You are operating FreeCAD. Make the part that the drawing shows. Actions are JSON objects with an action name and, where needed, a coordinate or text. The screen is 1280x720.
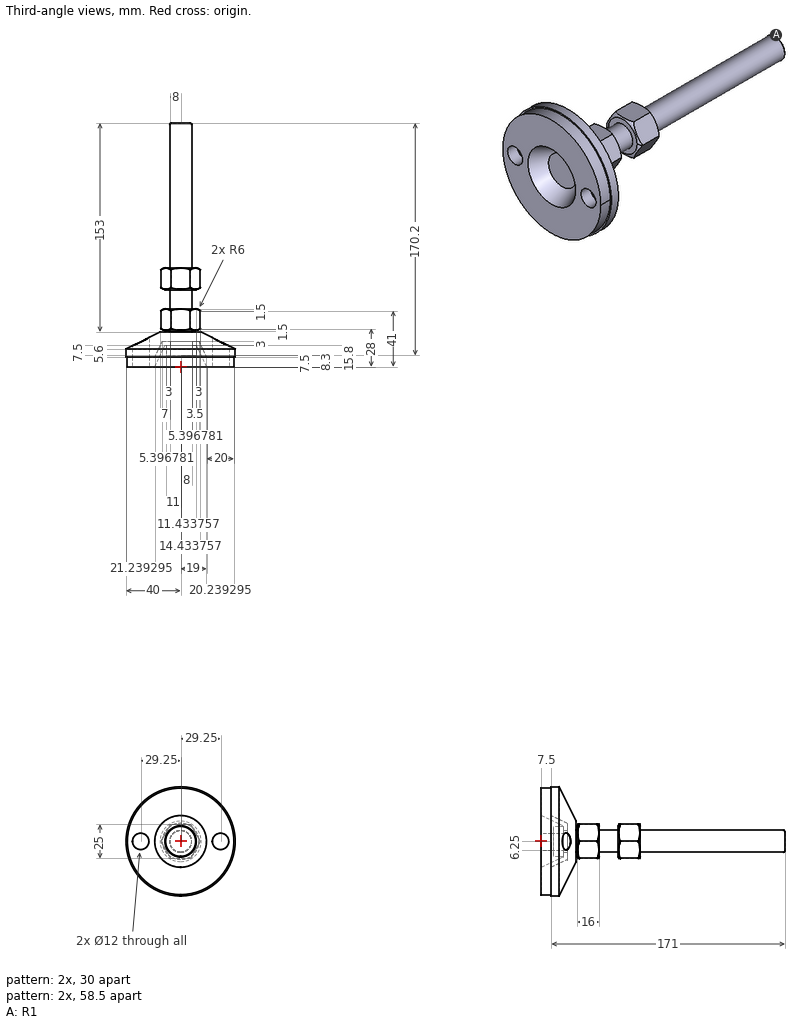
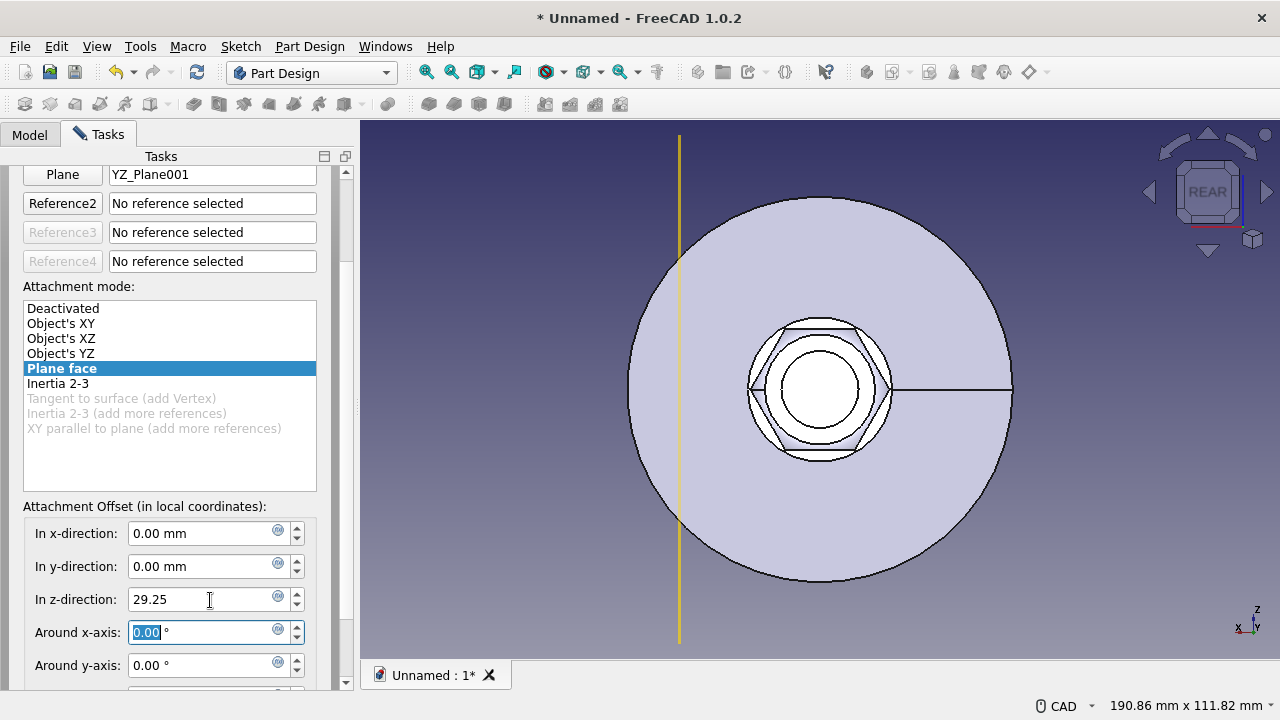
{"action": "scroll", "coordinate": [346, 428], "scroll_direction": "up", "scroll_amount": 3}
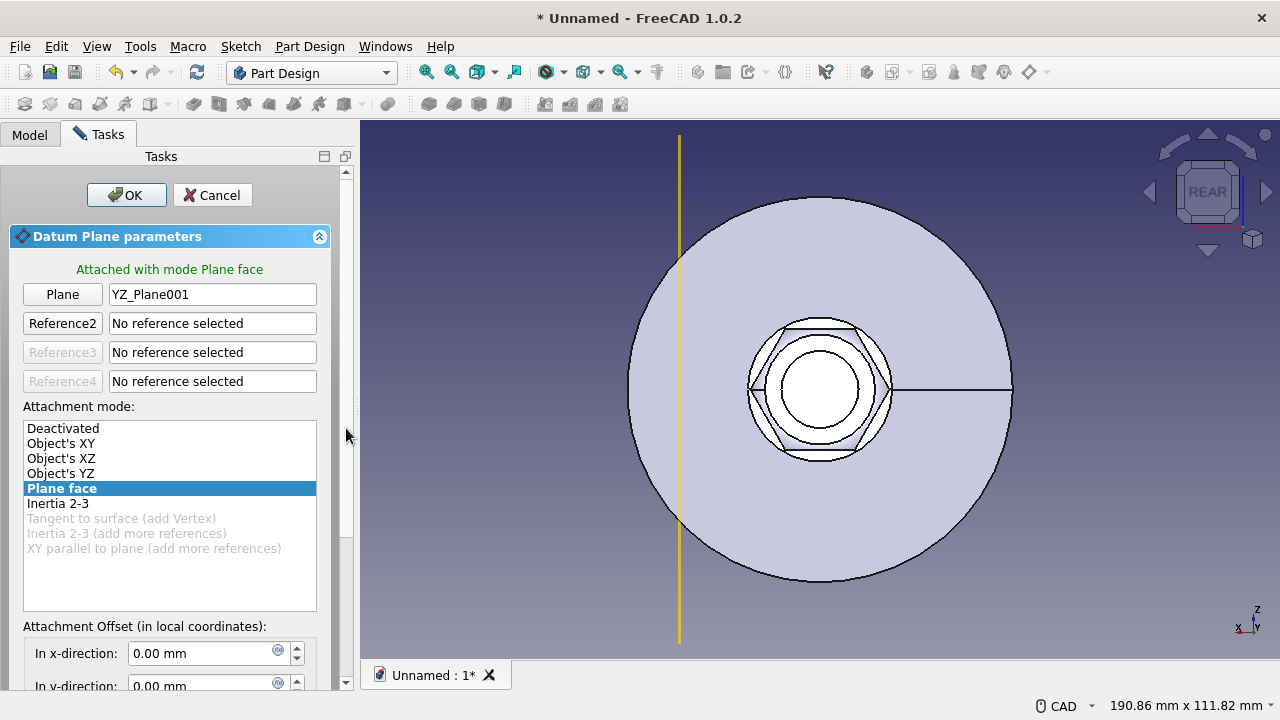
{"action": "left_click", "coordinate": [127, 195]}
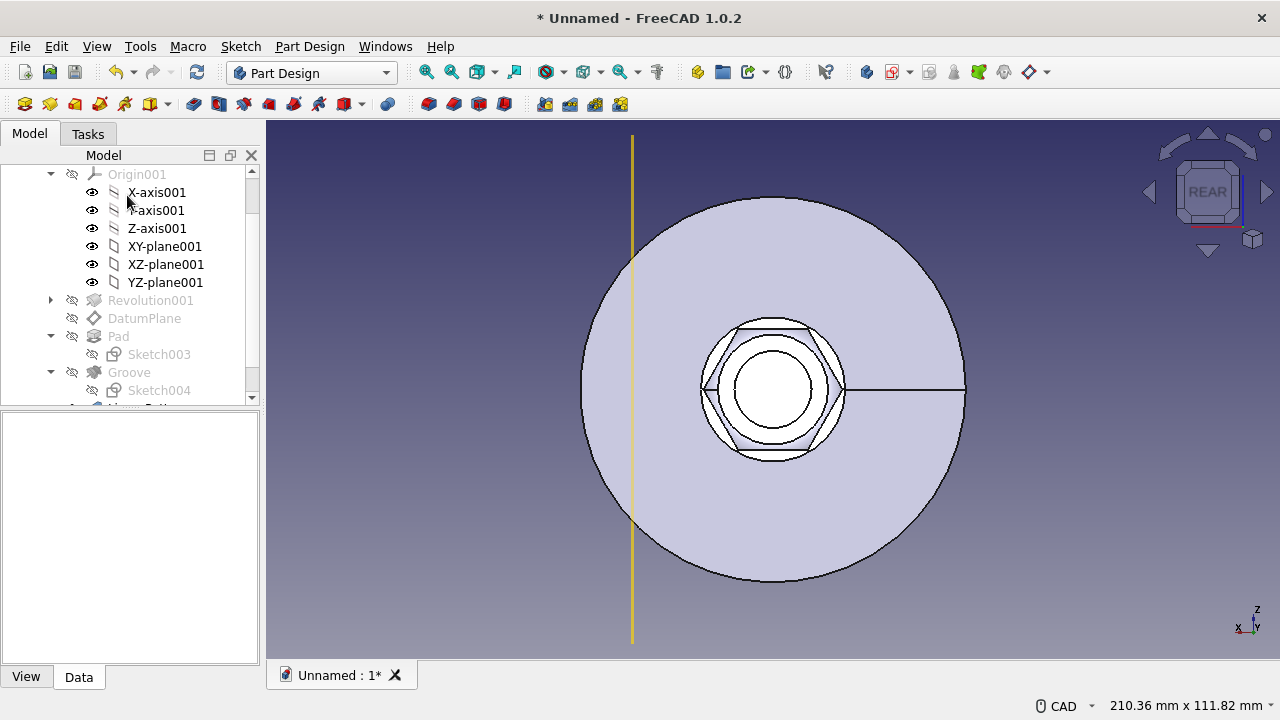
{"action": "scroll", "coordinate": [141, 278], "scroll_direction": "down", "scroll_amount": 3}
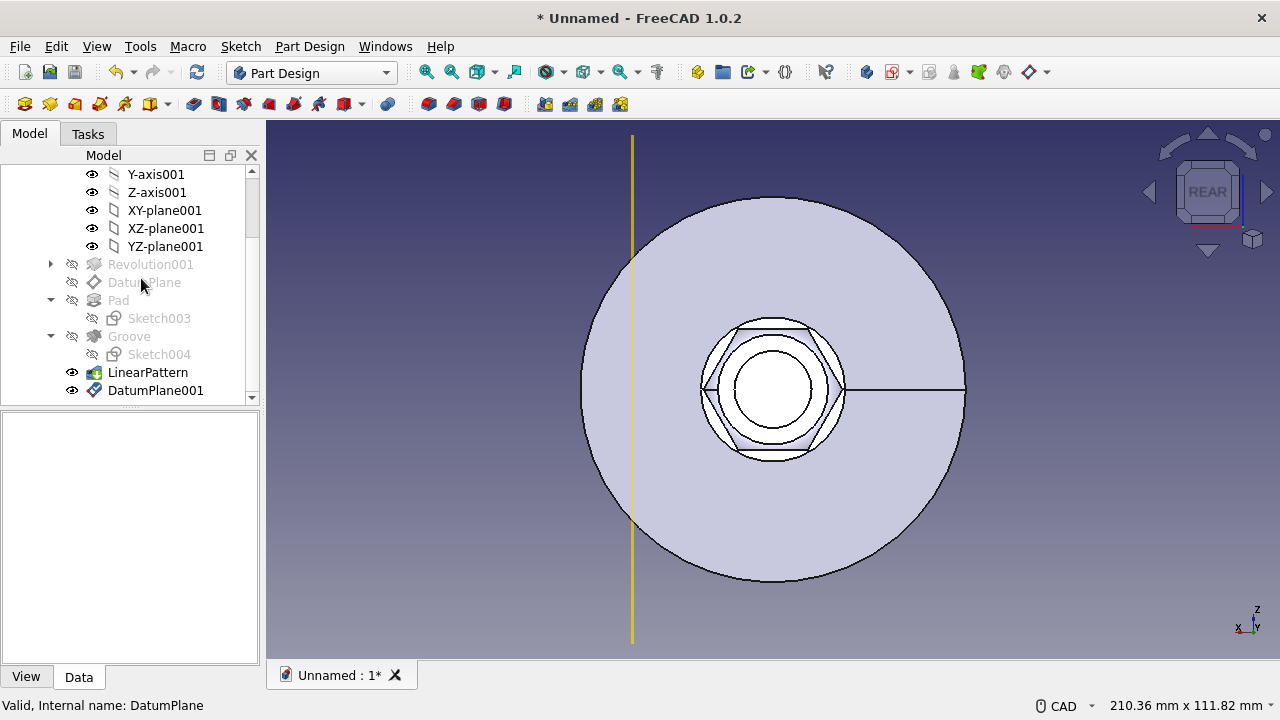
{"action": "left_click", "coordinate": [117, 390]}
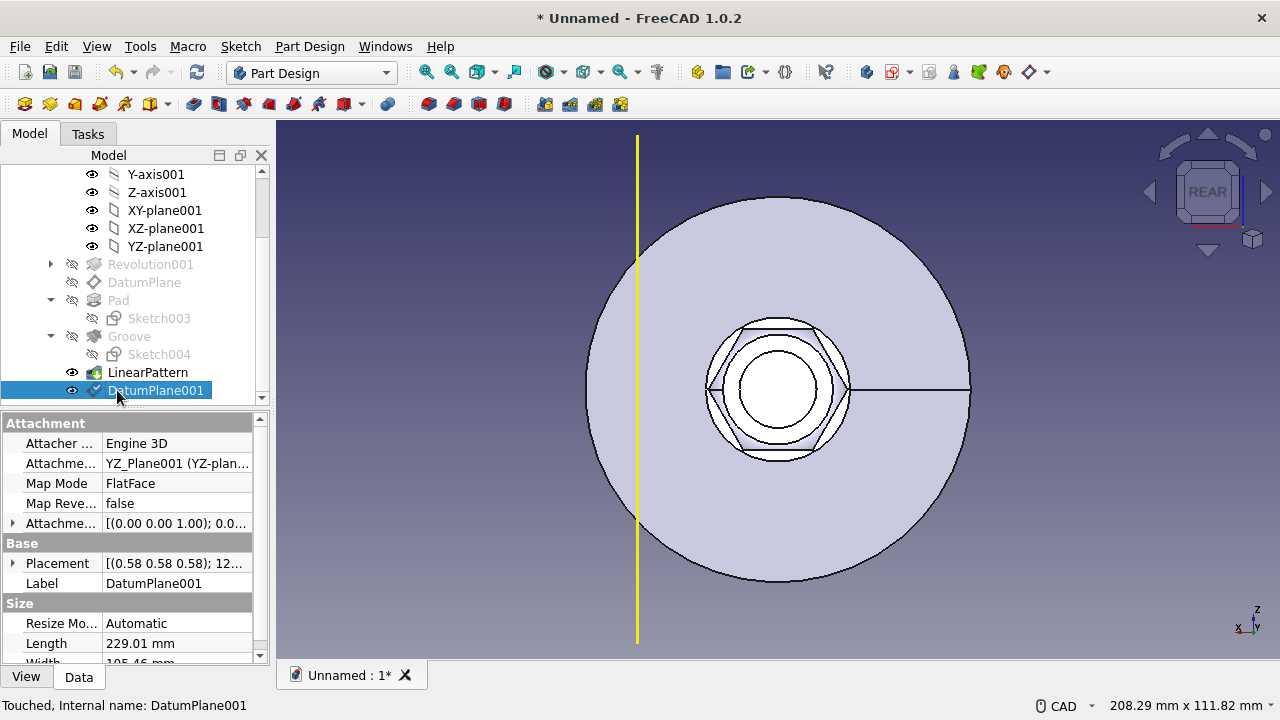
{"action": "left_click", "coordinate": [892, 72]}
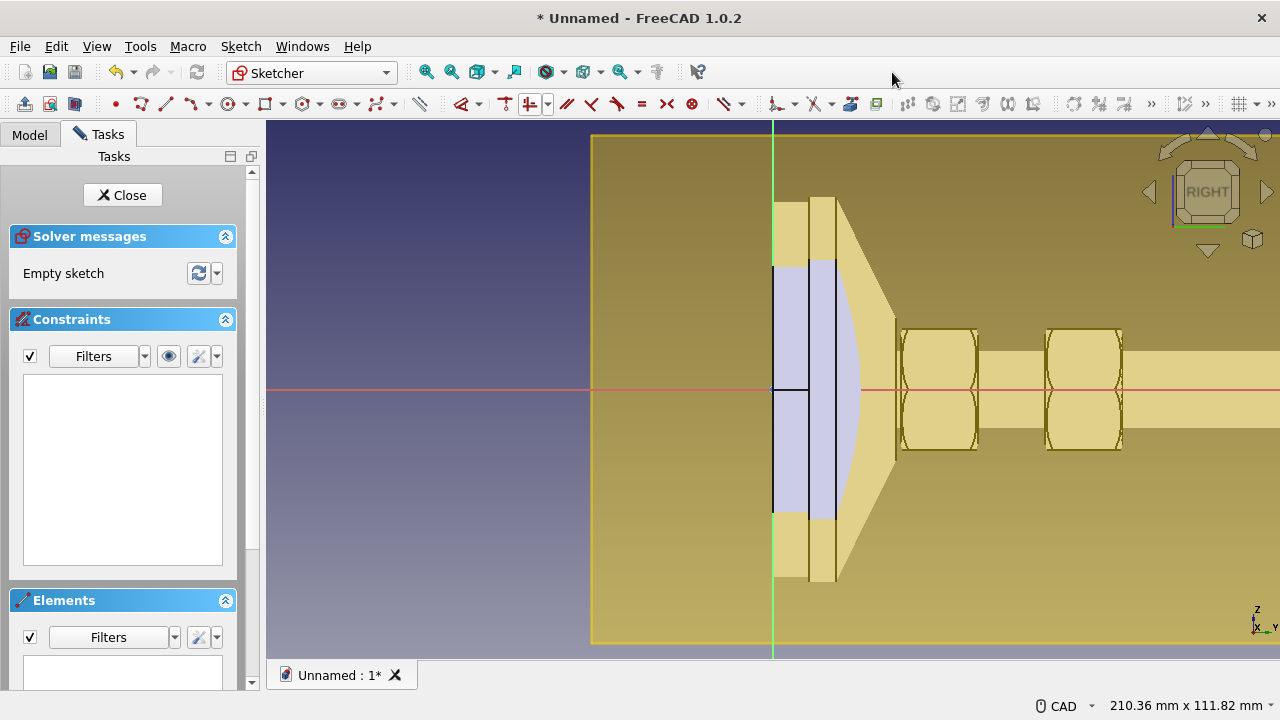
{"action": "left_click", "coordinate": [75, 104]}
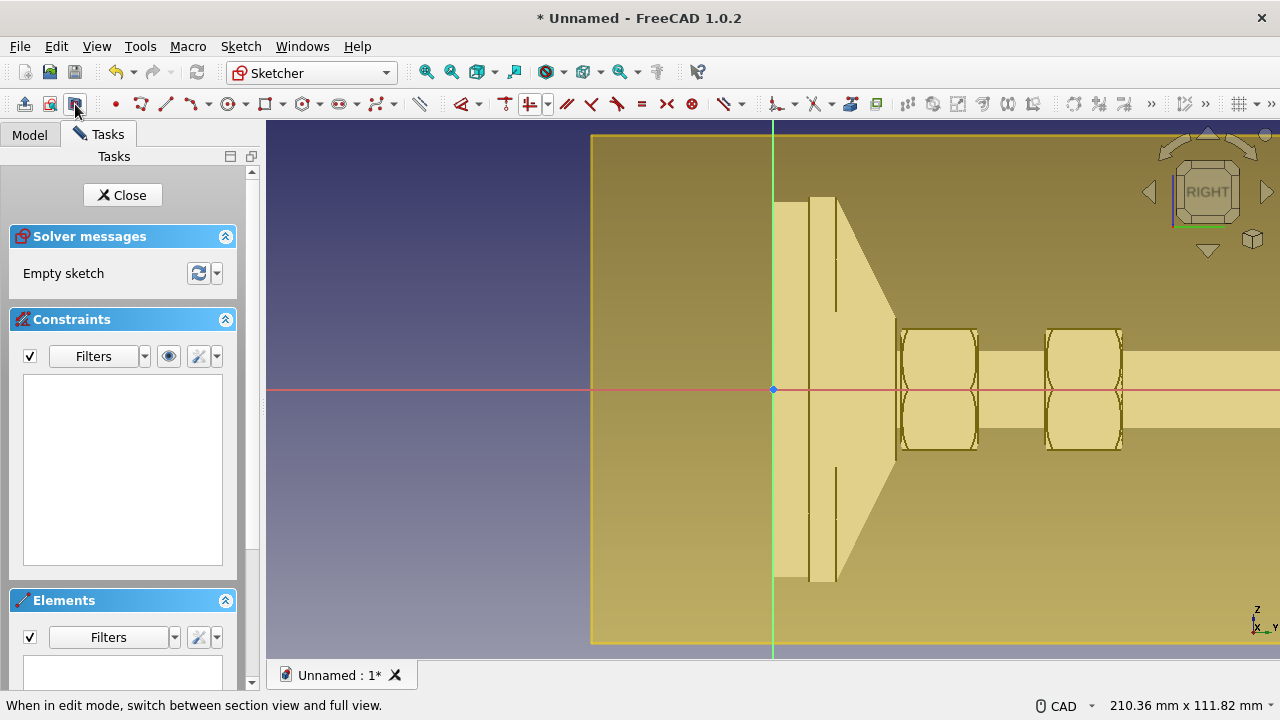
{"action": "scroll", "coordinate": [294, 371], "scroll_direction": "down", "scroll_amount": 3}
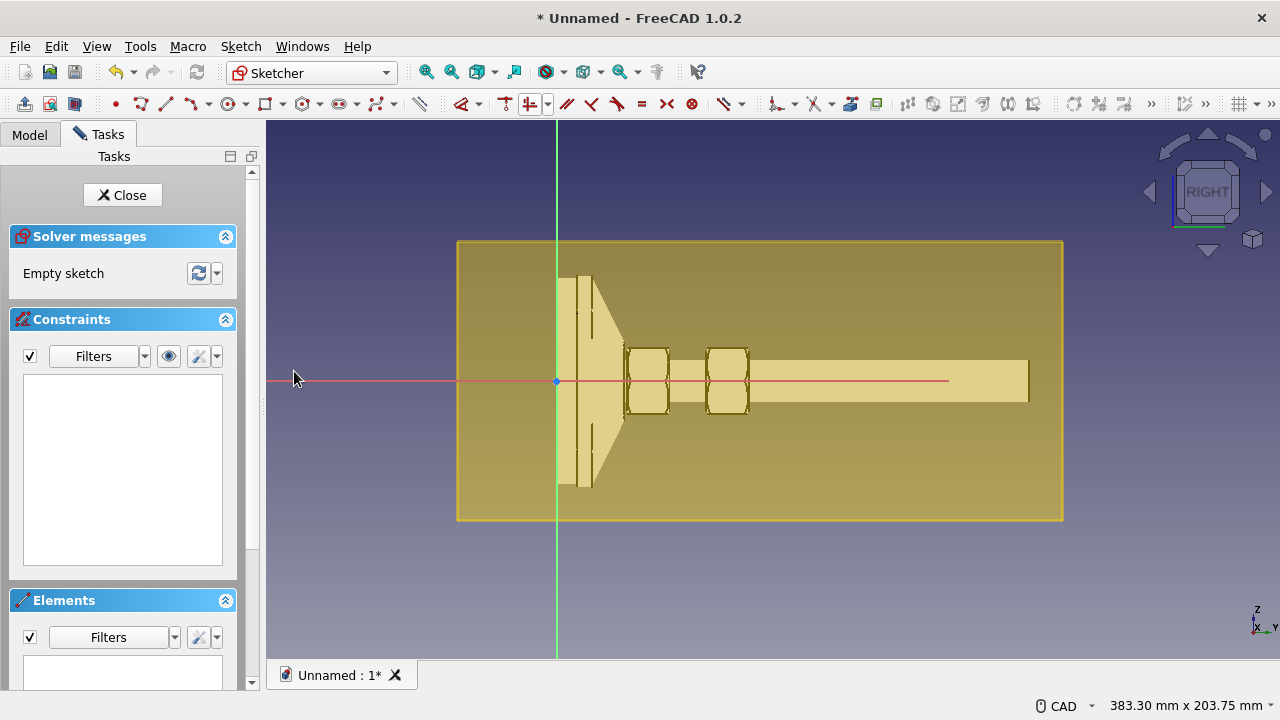
{"action": "left_click", "coordinate": [264, 104]}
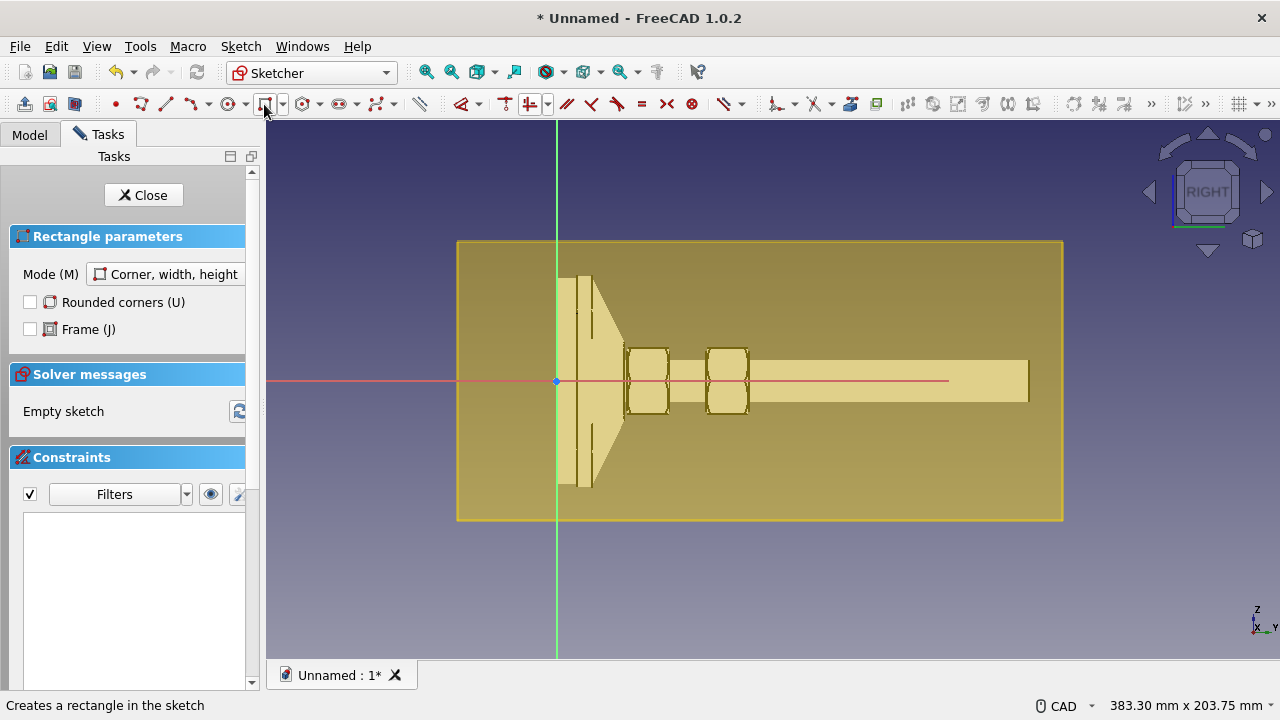
{"action": "left_click", "coordinate": [577, 381]}
{"action": "left_click", "coordinate": [1029, 398]}
{"action": "key", "text": "Escape"}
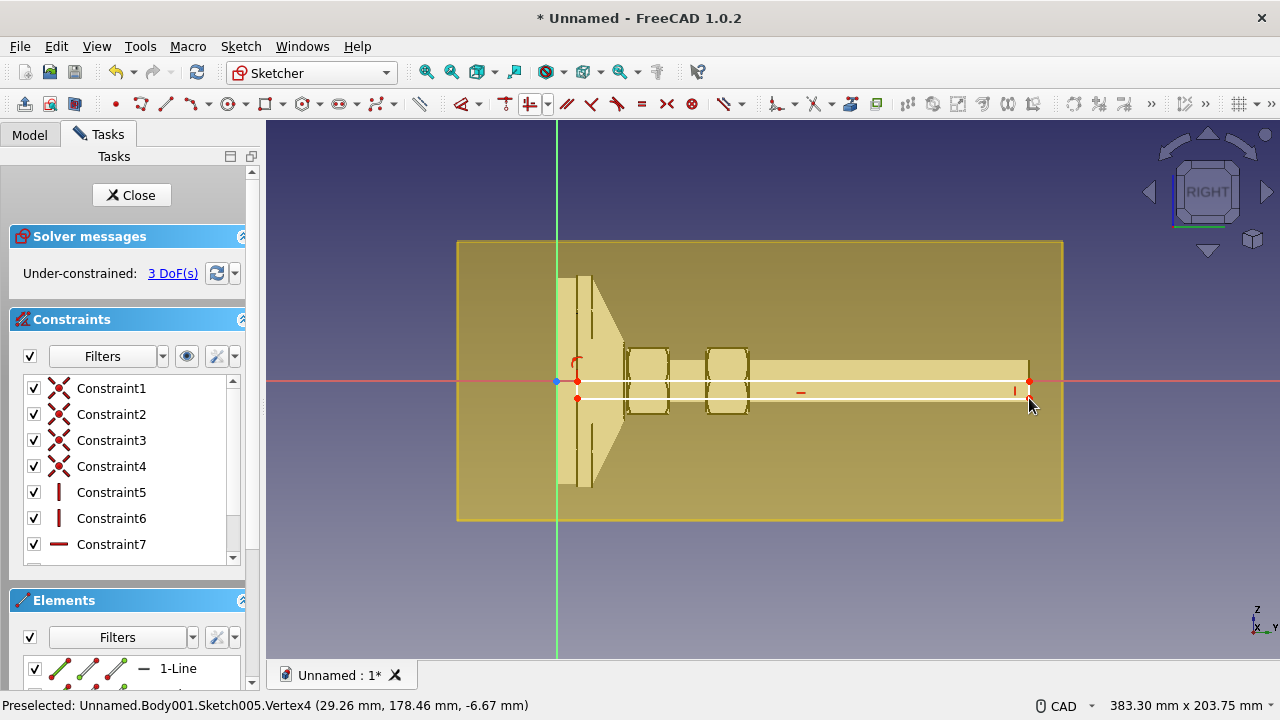
{"action": "left_click", "coordinate": [460, 104]}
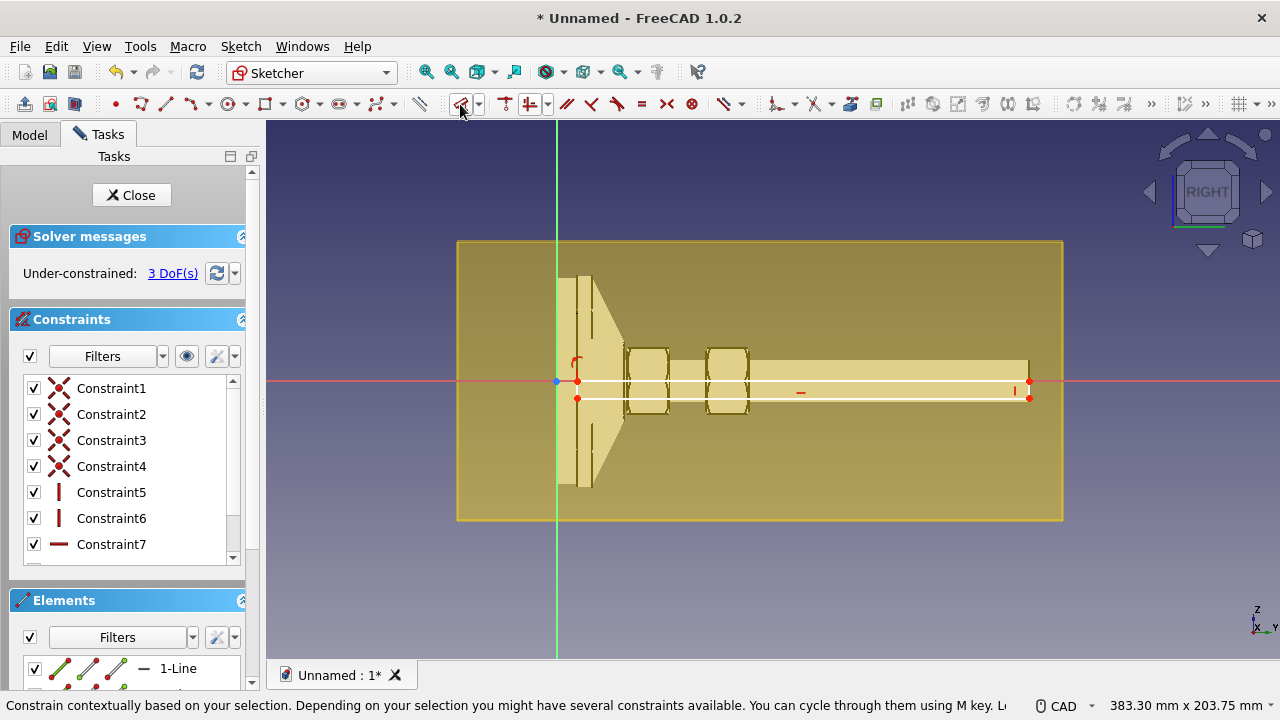
{"action": "left_click", "coordinate": [713, 399]}
{"action": "left_click", "coordinate": [803, 433]}